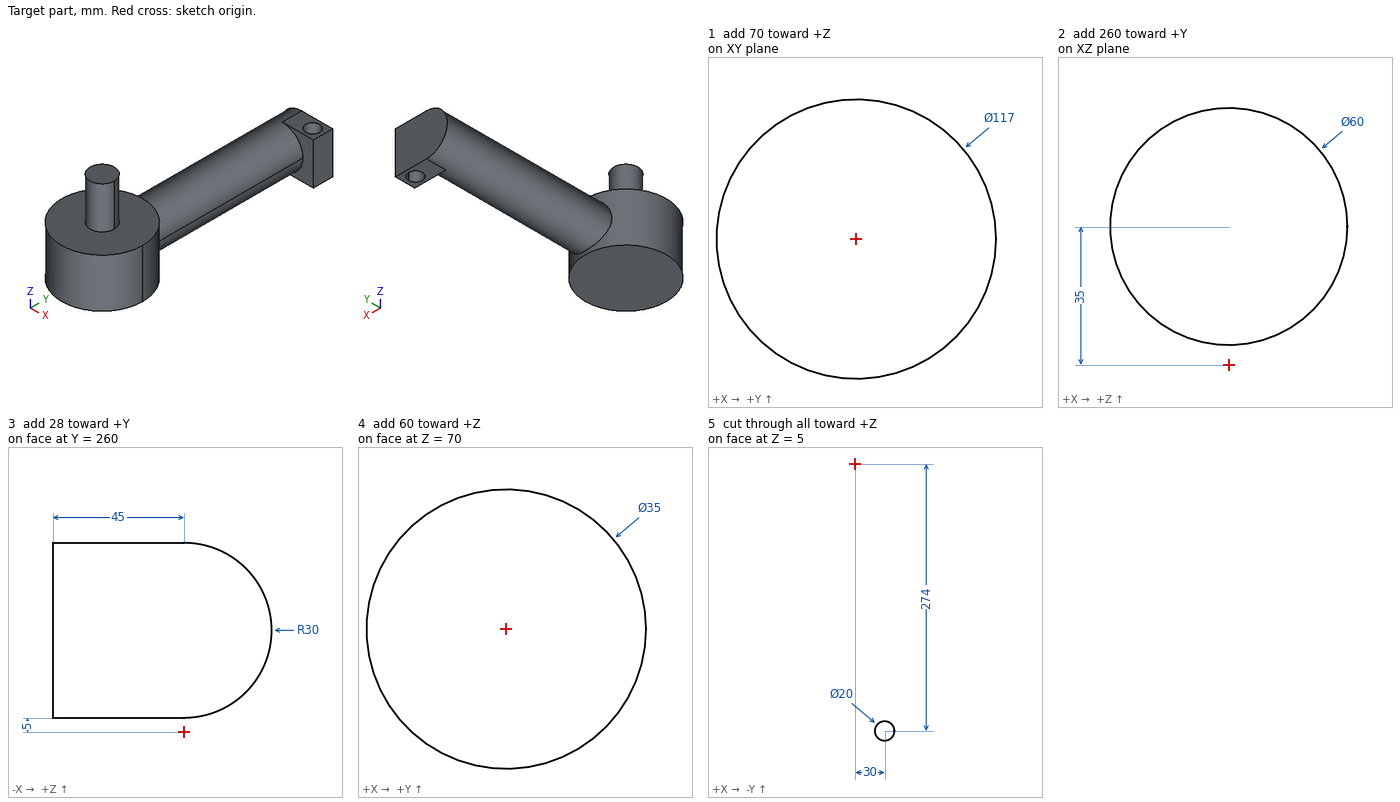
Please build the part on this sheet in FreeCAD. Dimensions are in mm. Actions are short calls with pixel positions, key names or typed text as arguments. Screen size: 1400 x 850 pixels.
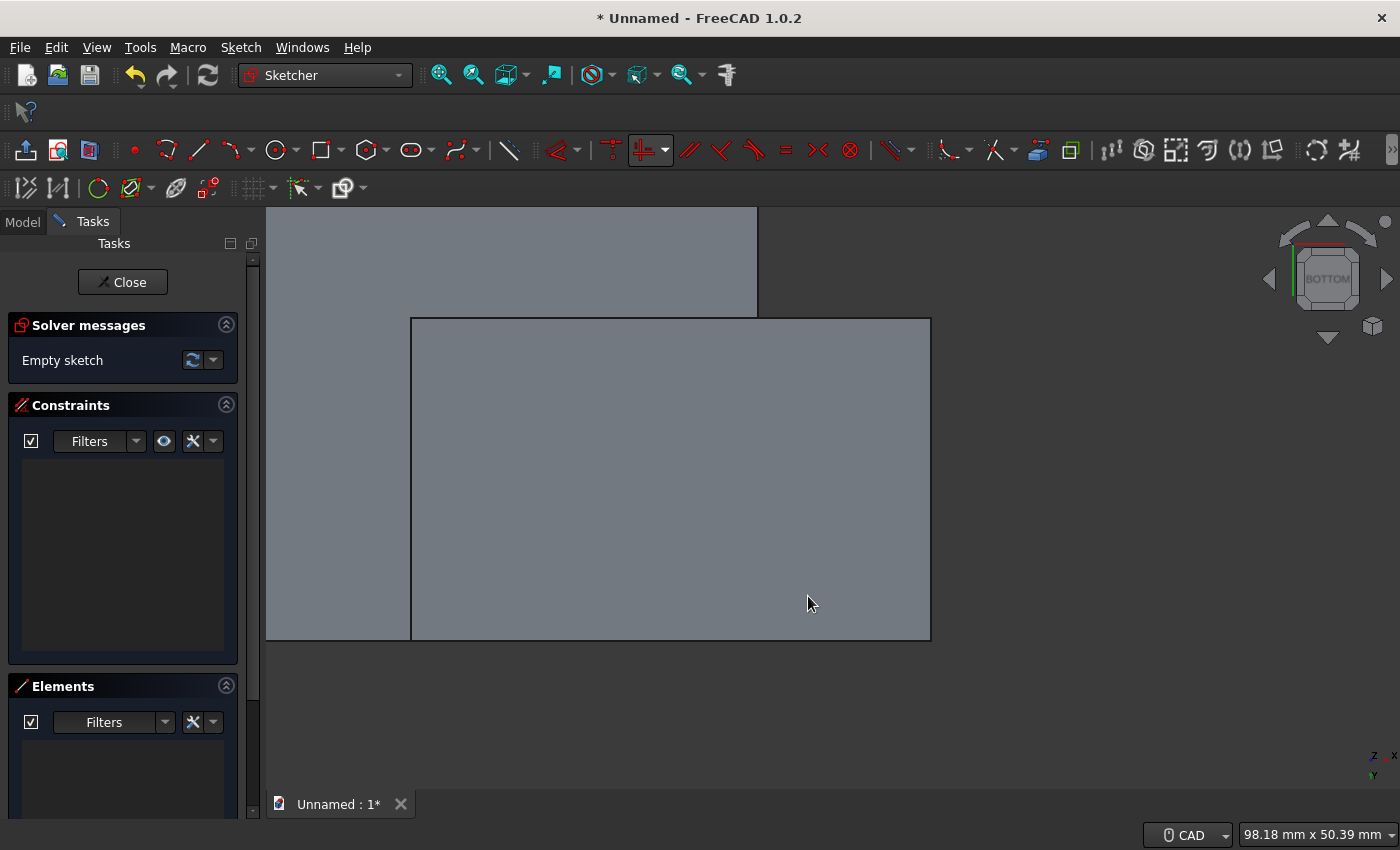
scroll(744, 442, up, 2)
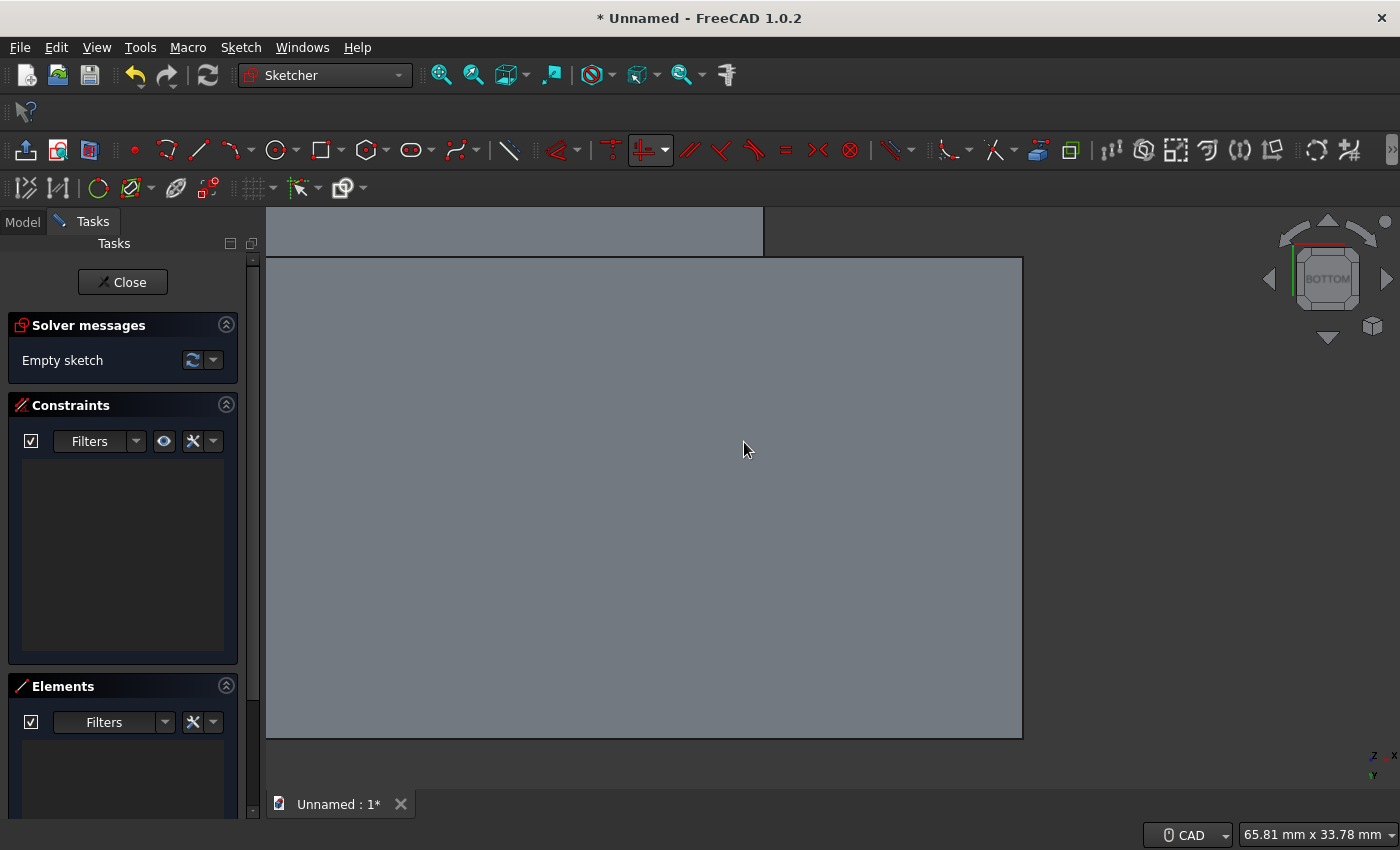
key(g)
key(c)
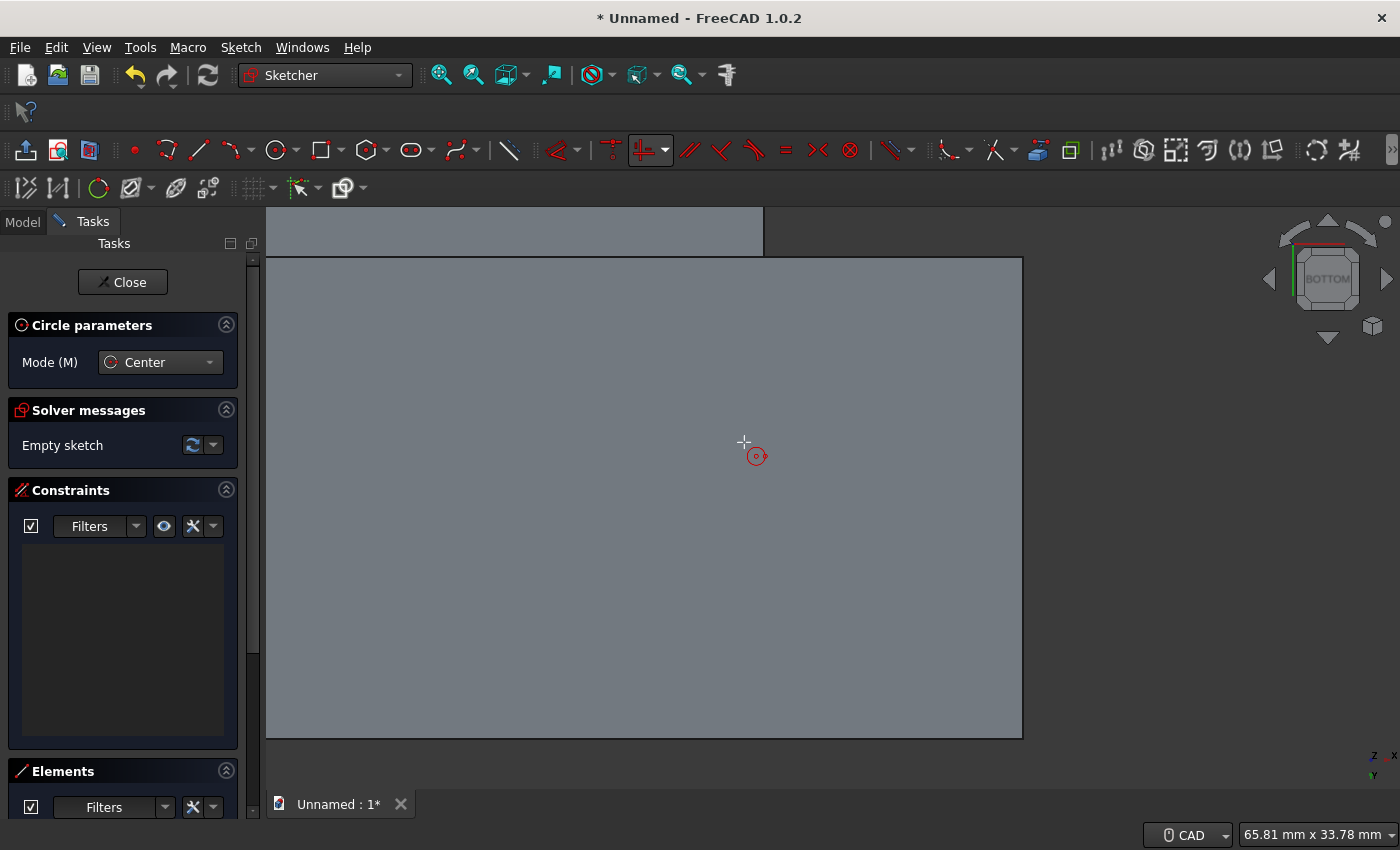
click(764, 498)
click(886, 376)
key(Escape)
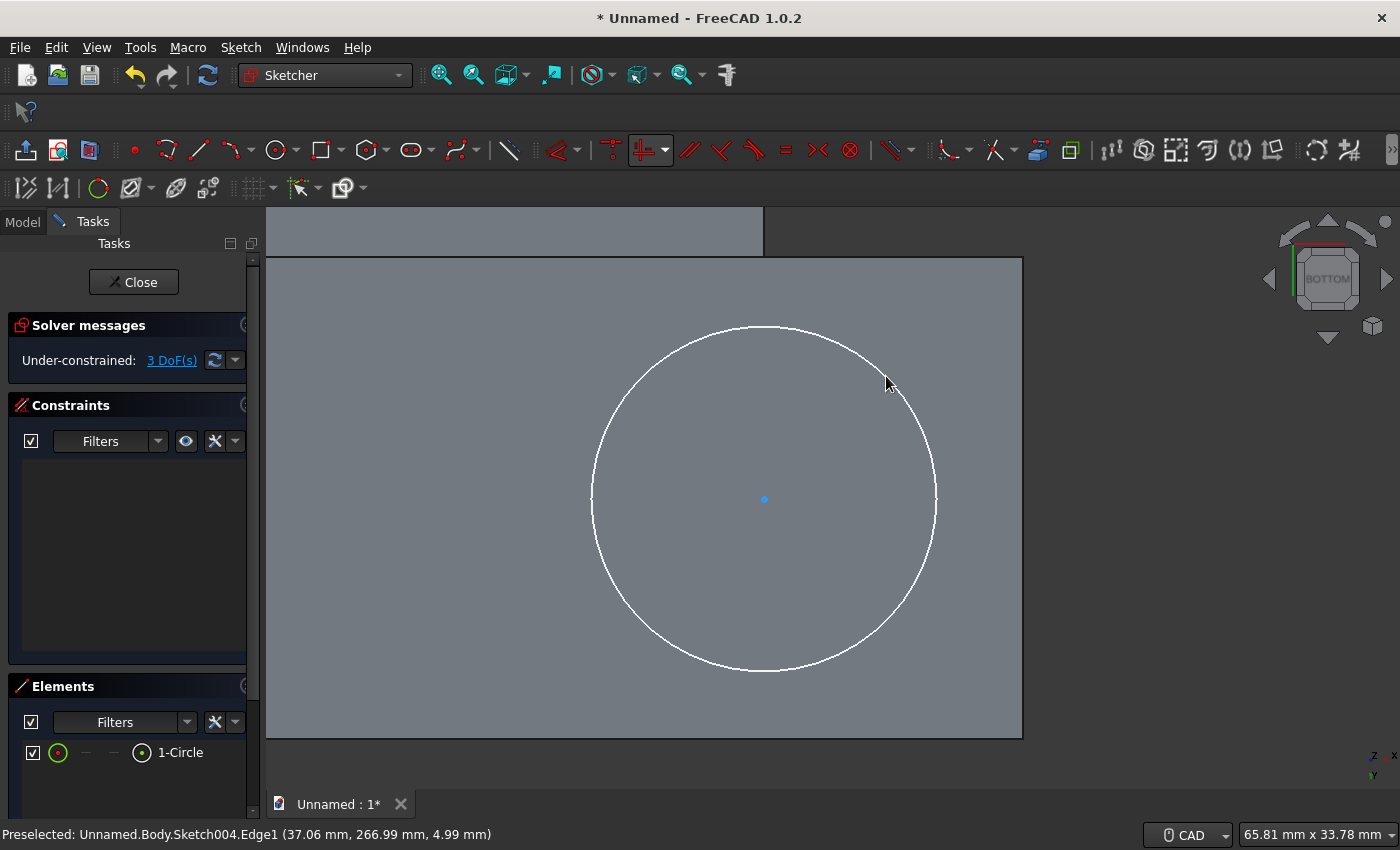
key(d)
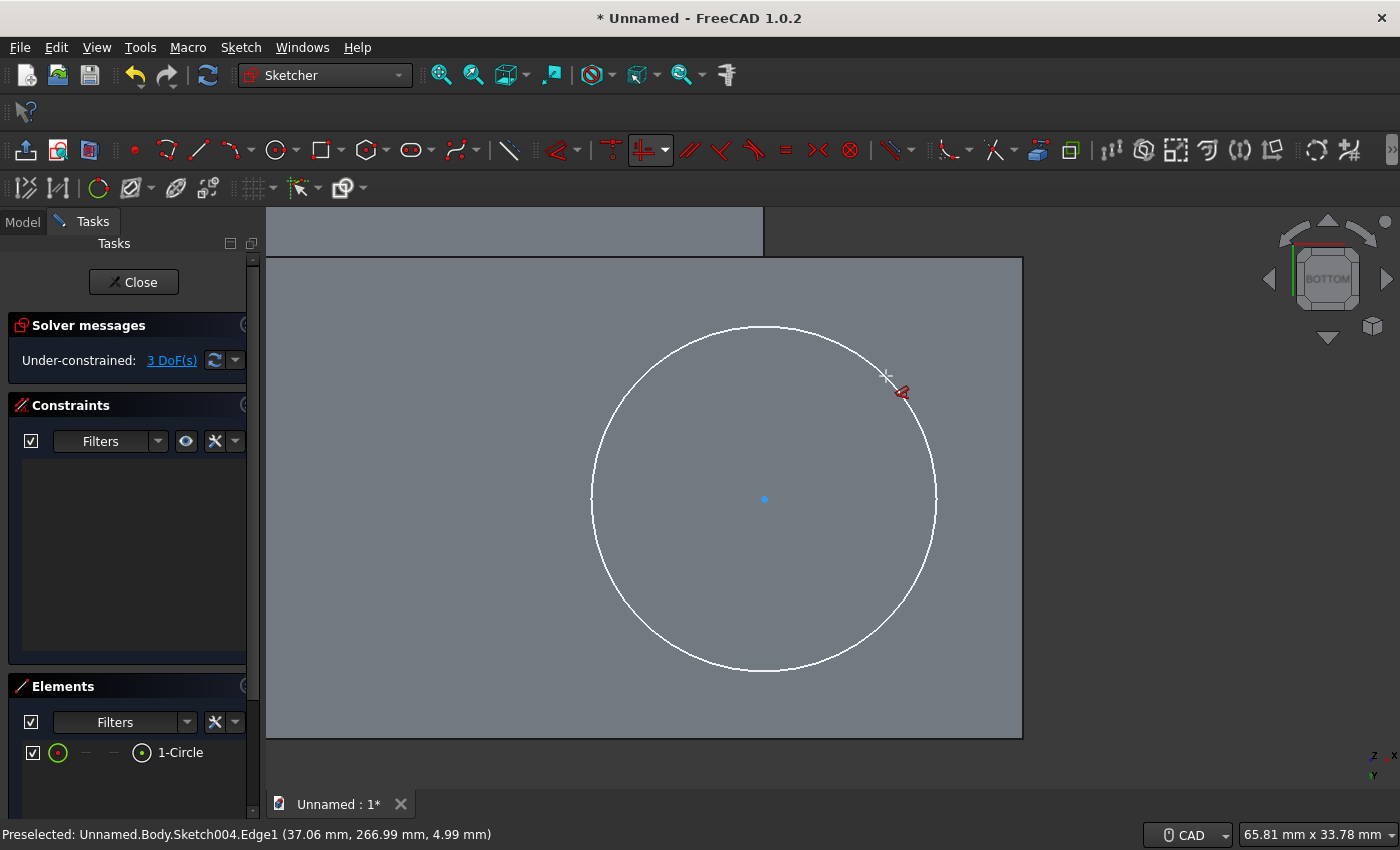
click(886, 377)
click(909, 354)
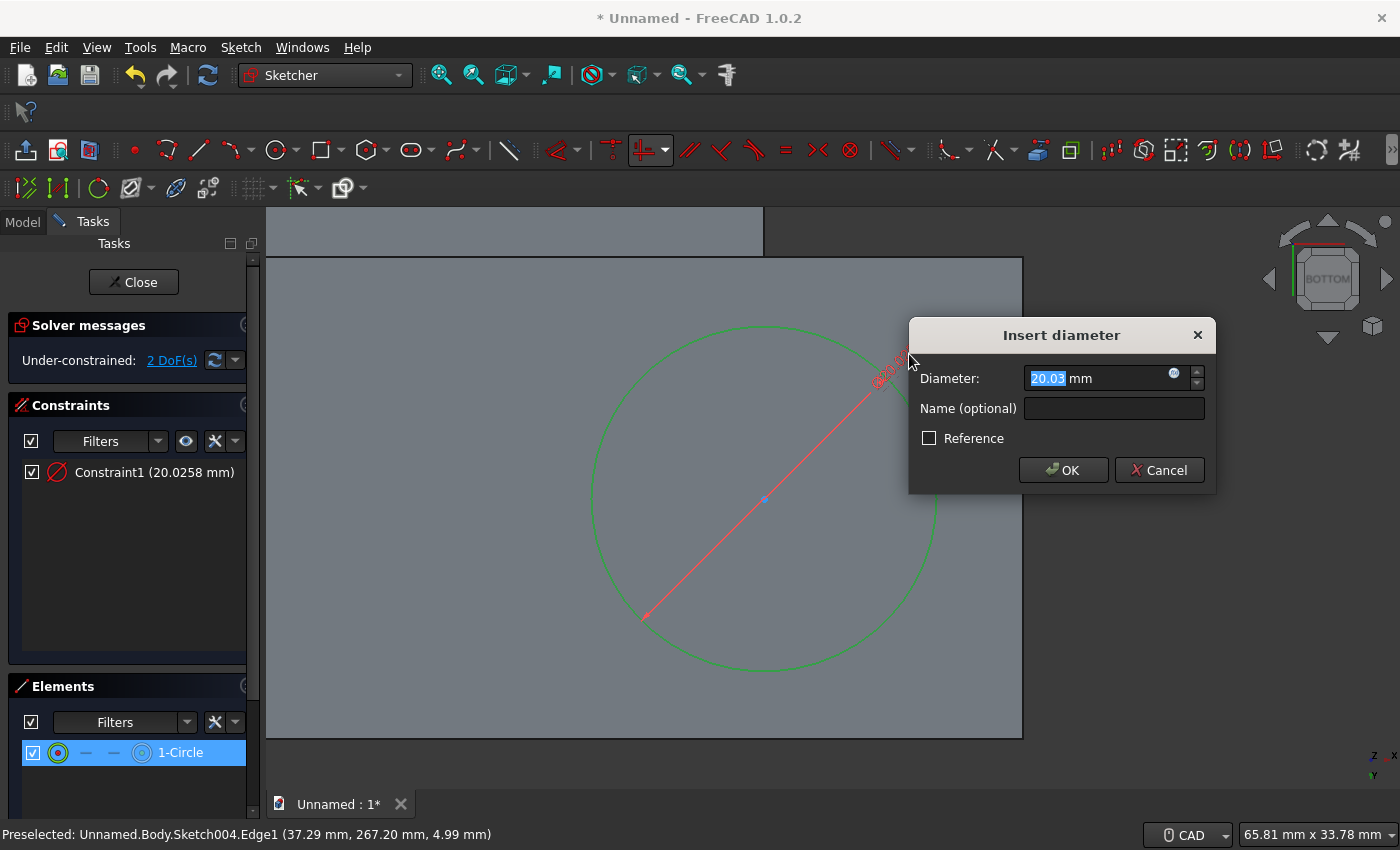
text(20)
key(Return)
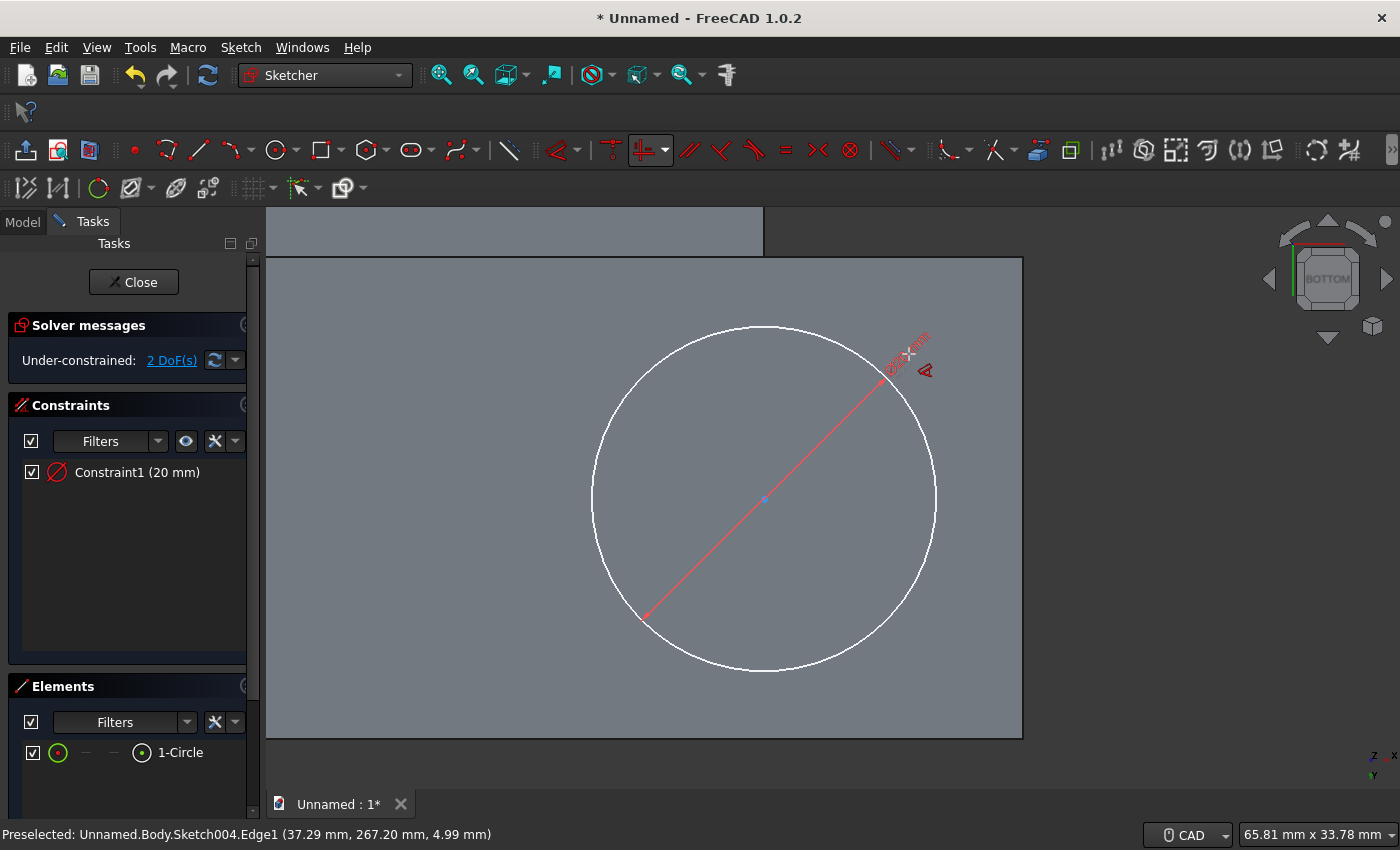
click(764, 499)
click(529, 533)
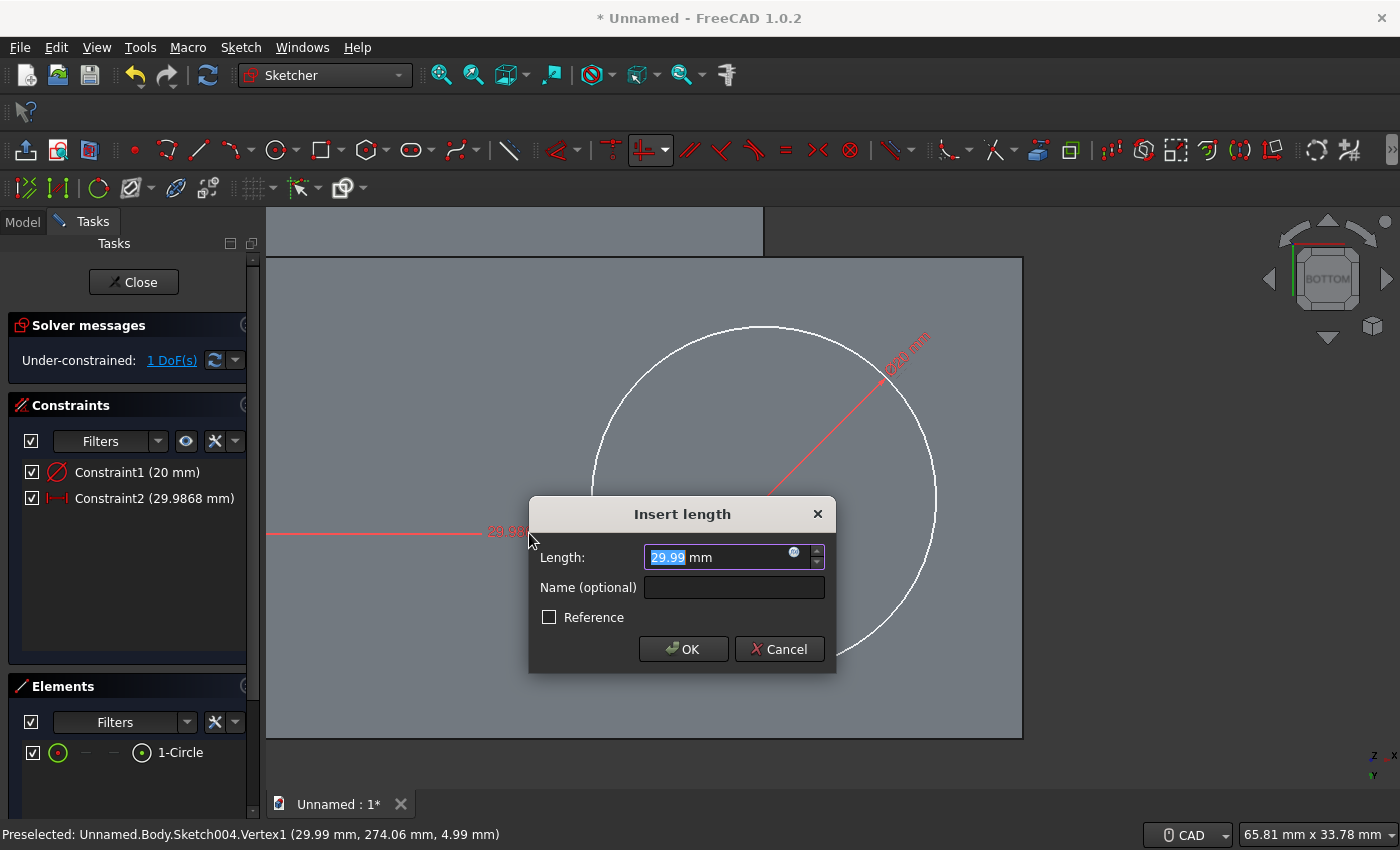
text(30)
key(Return)